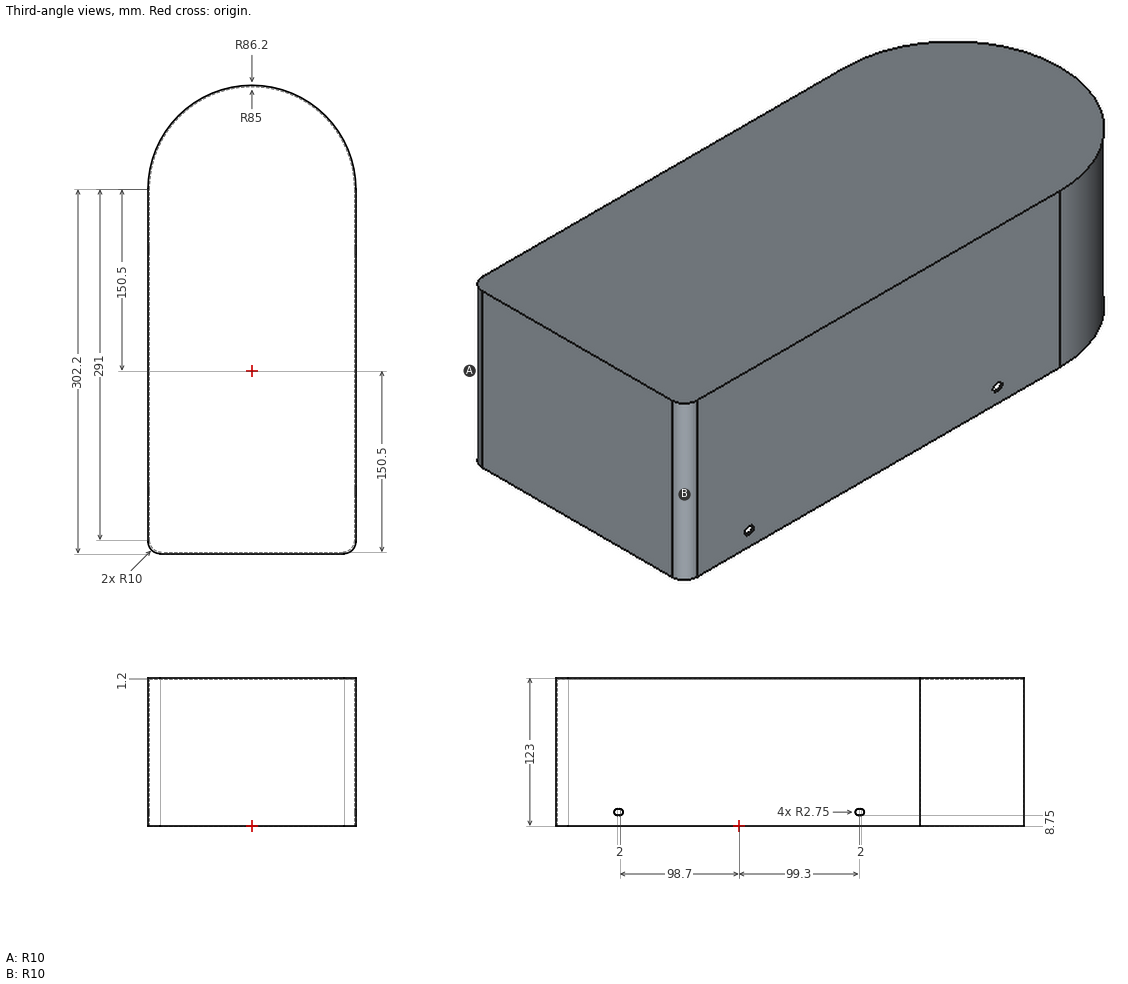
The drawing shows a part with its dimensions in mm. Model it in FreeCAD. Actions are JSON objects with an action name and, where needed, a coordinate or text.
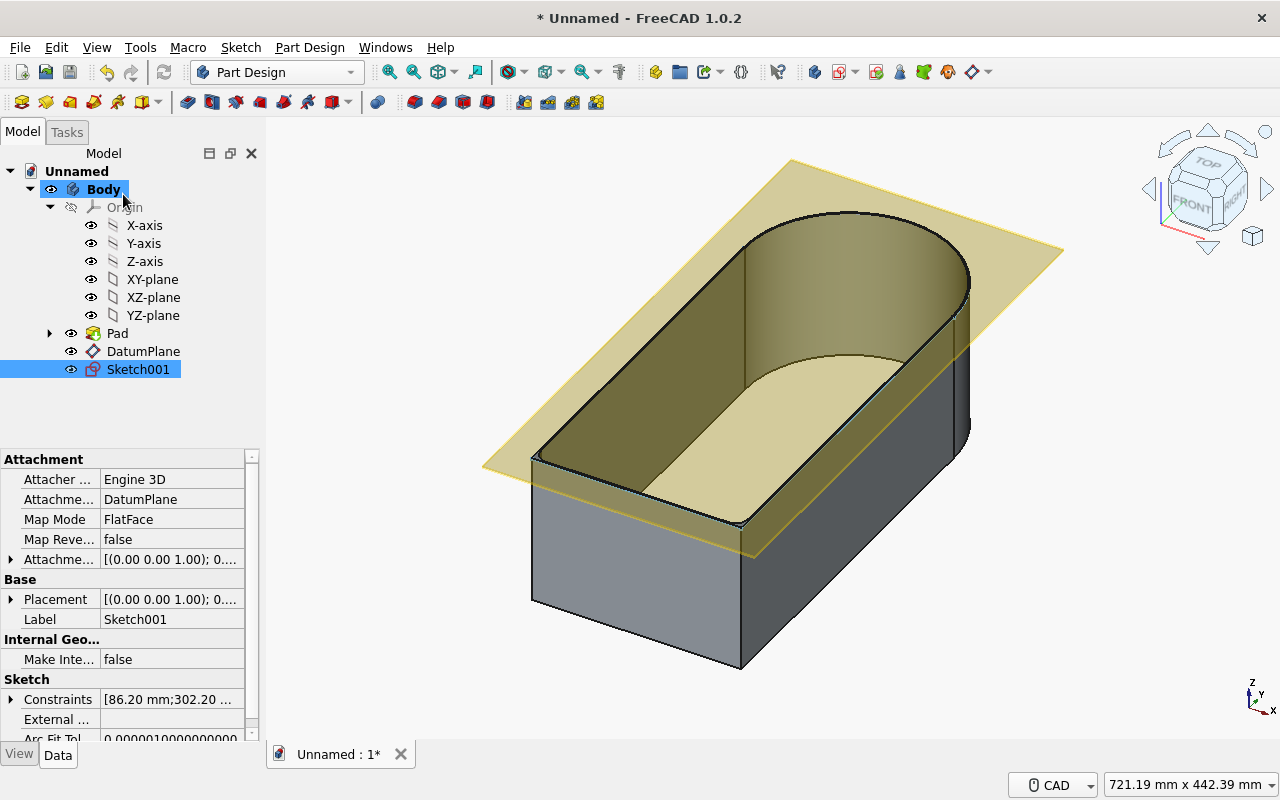
{"action": "left_click", "coordinate": [22, 102]}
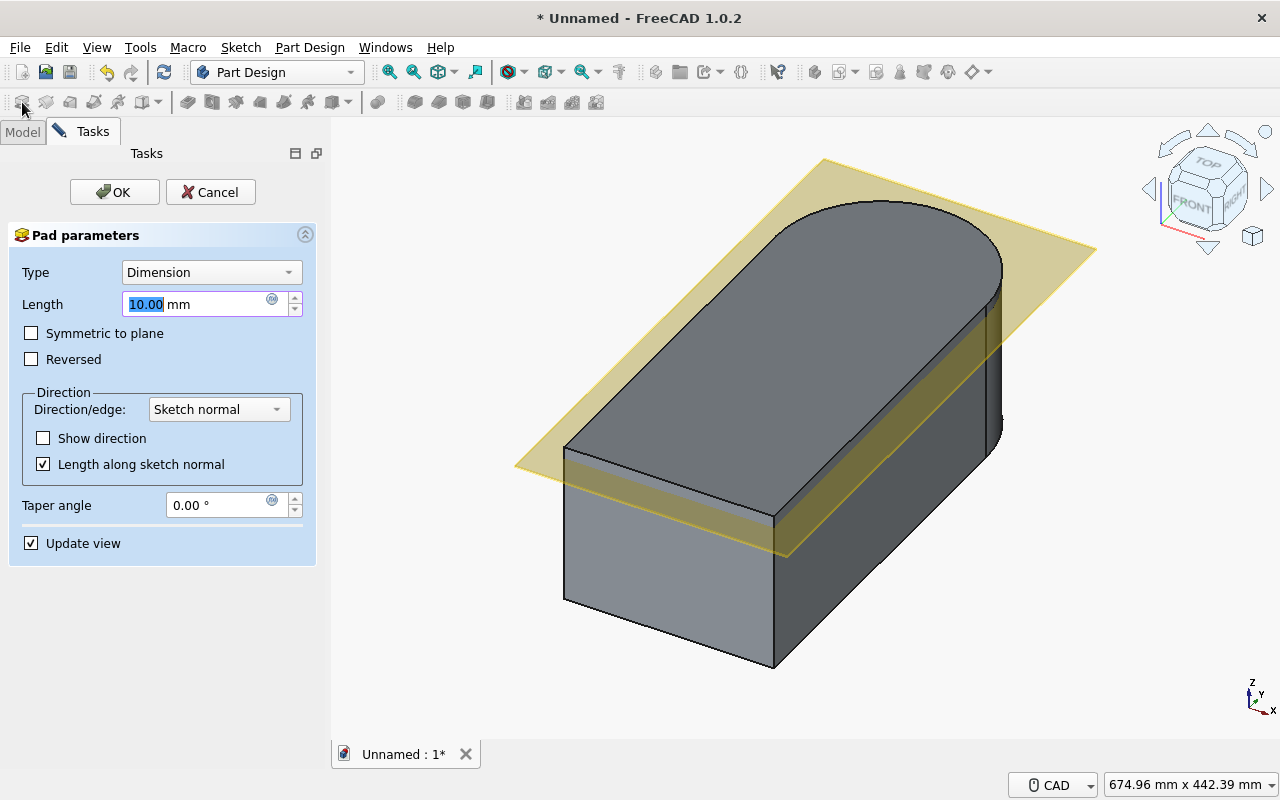
{"action": "type", "text": "1.2"}
{"action": "key", "text": "Tab"}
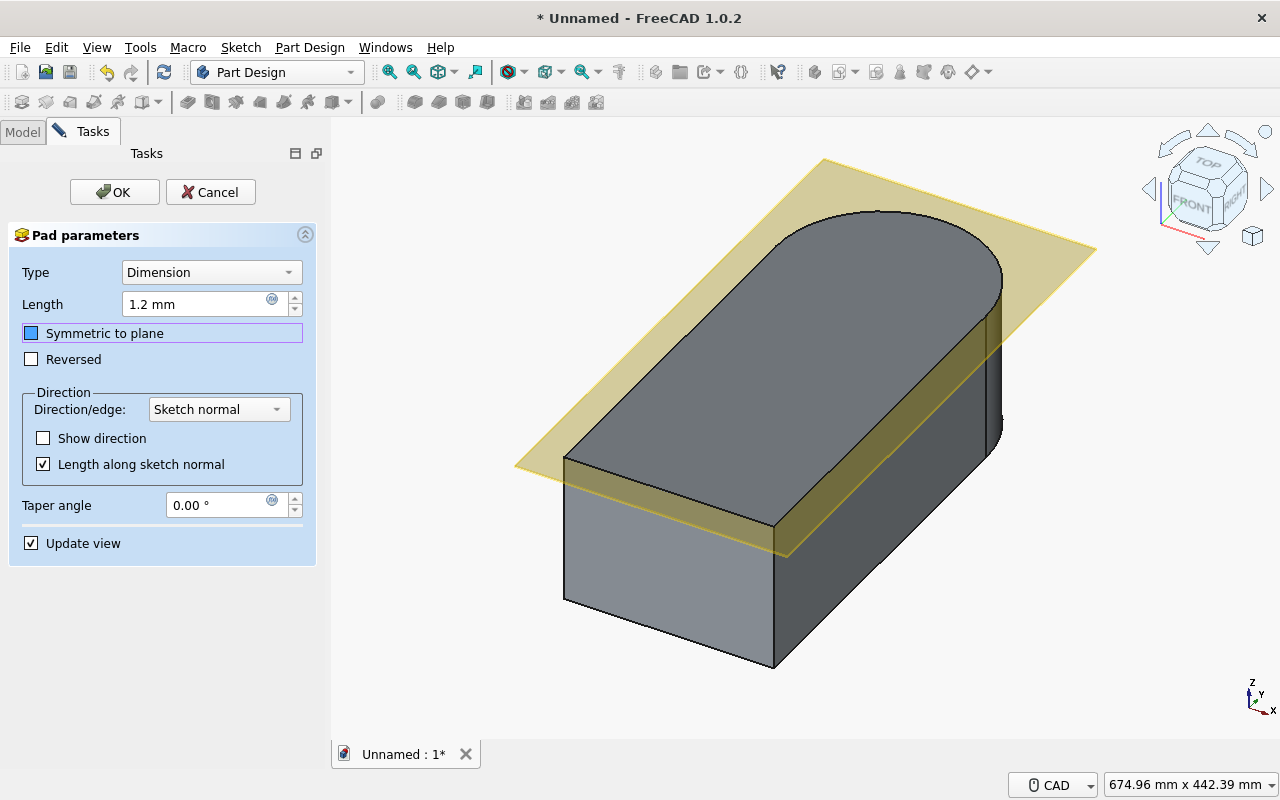
{"action": "left_click", "coordinate": [115, 192]}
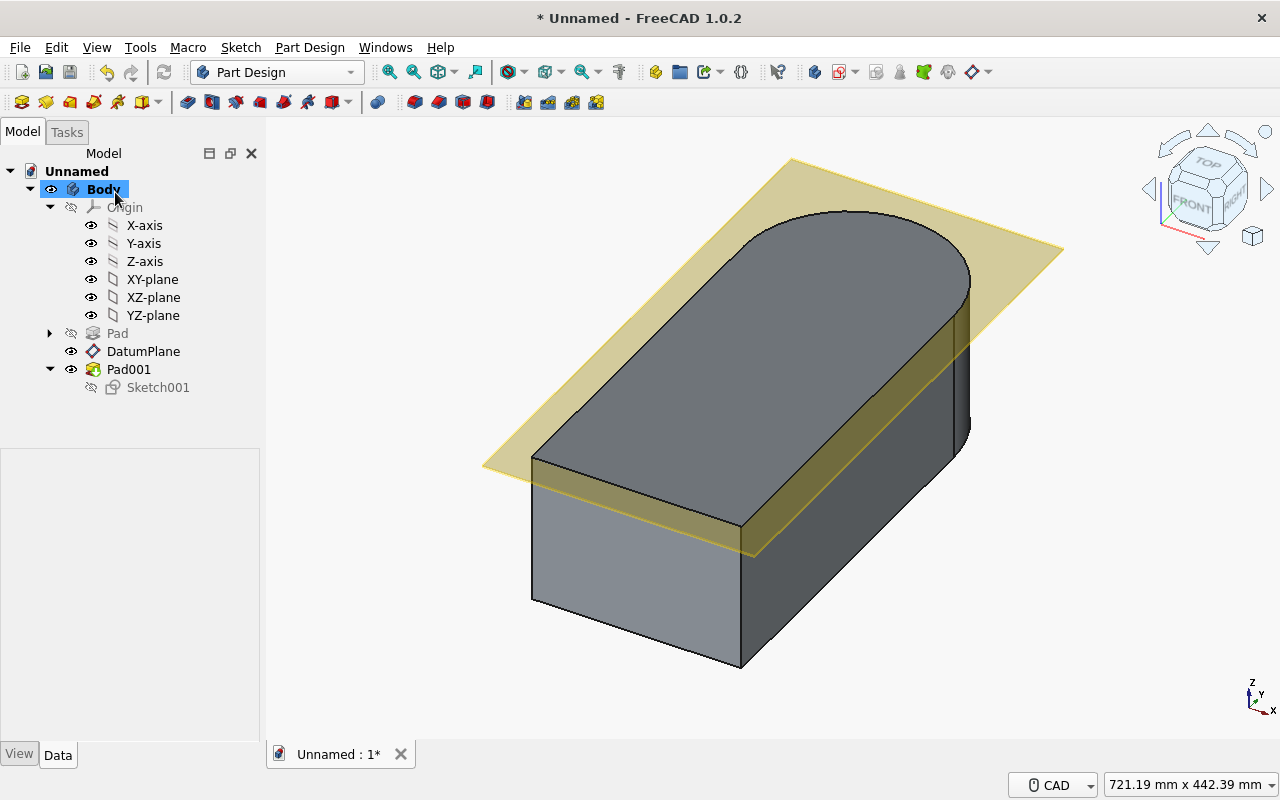
{"action": "left_click", "coordinate": [116, 351]}
{"action": "key", "text": "space"}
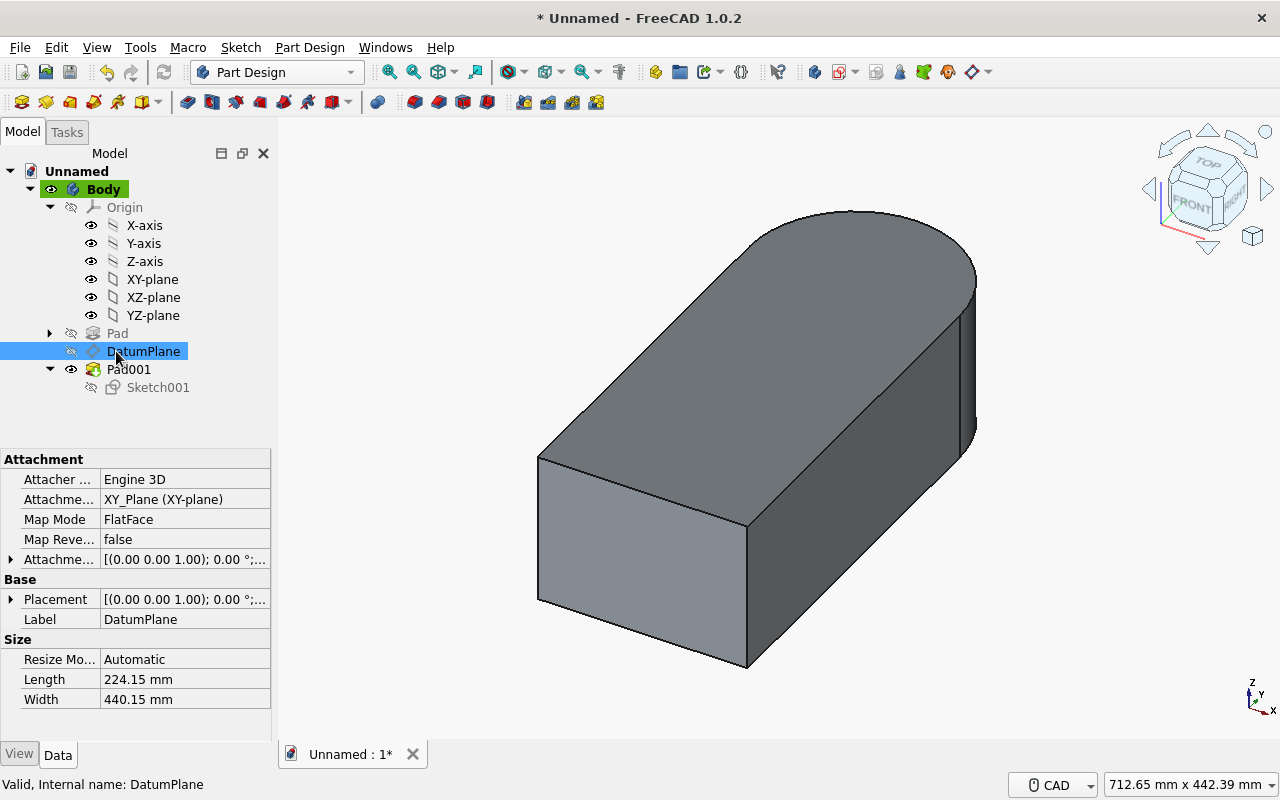
{"action": "key", "text": "0"}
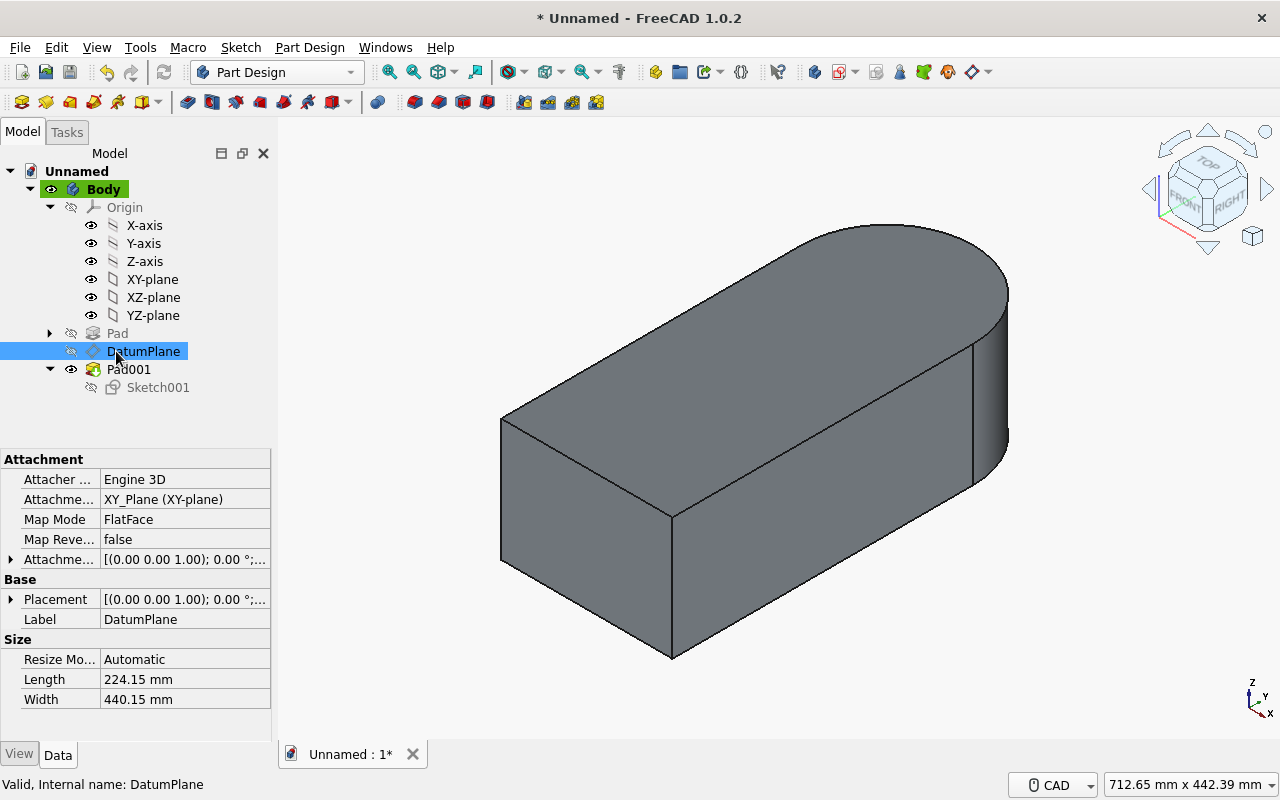
{"action": "key", "text": "2"}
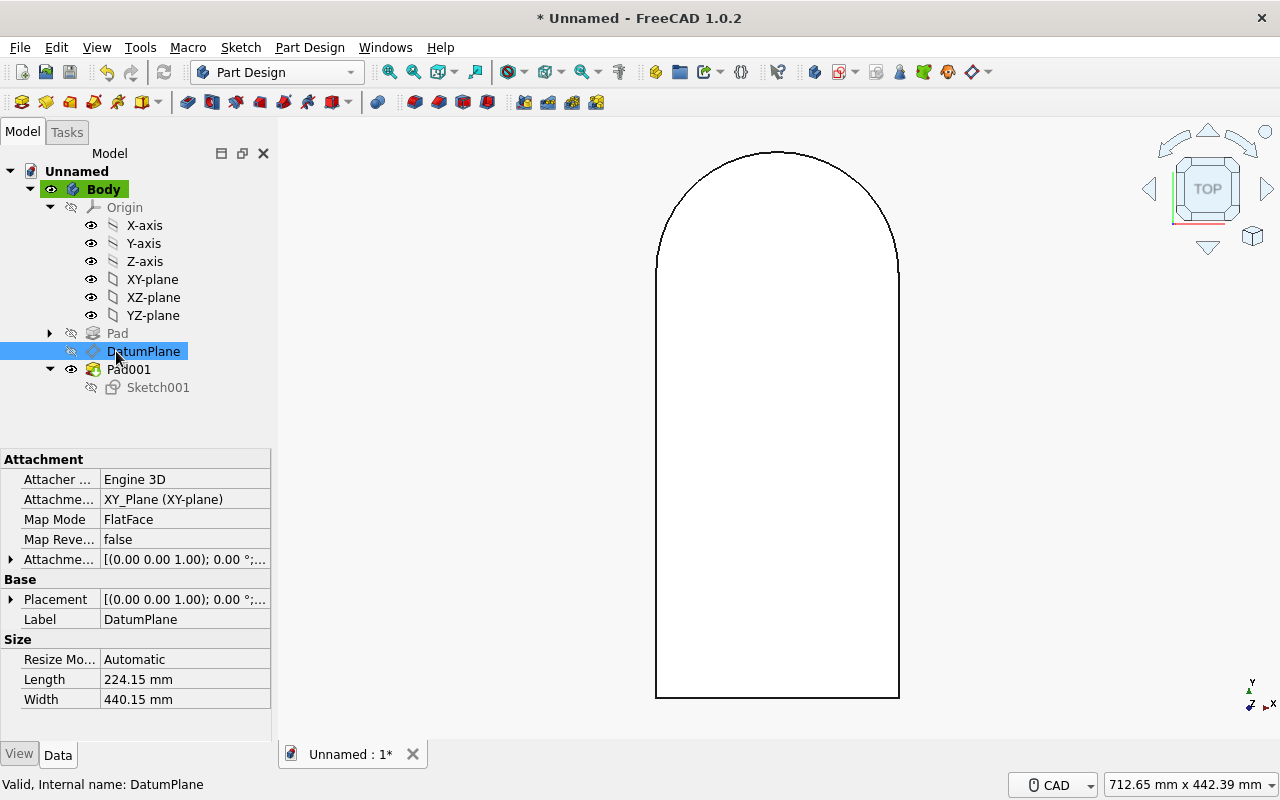
{"action": "key", "text": "1"}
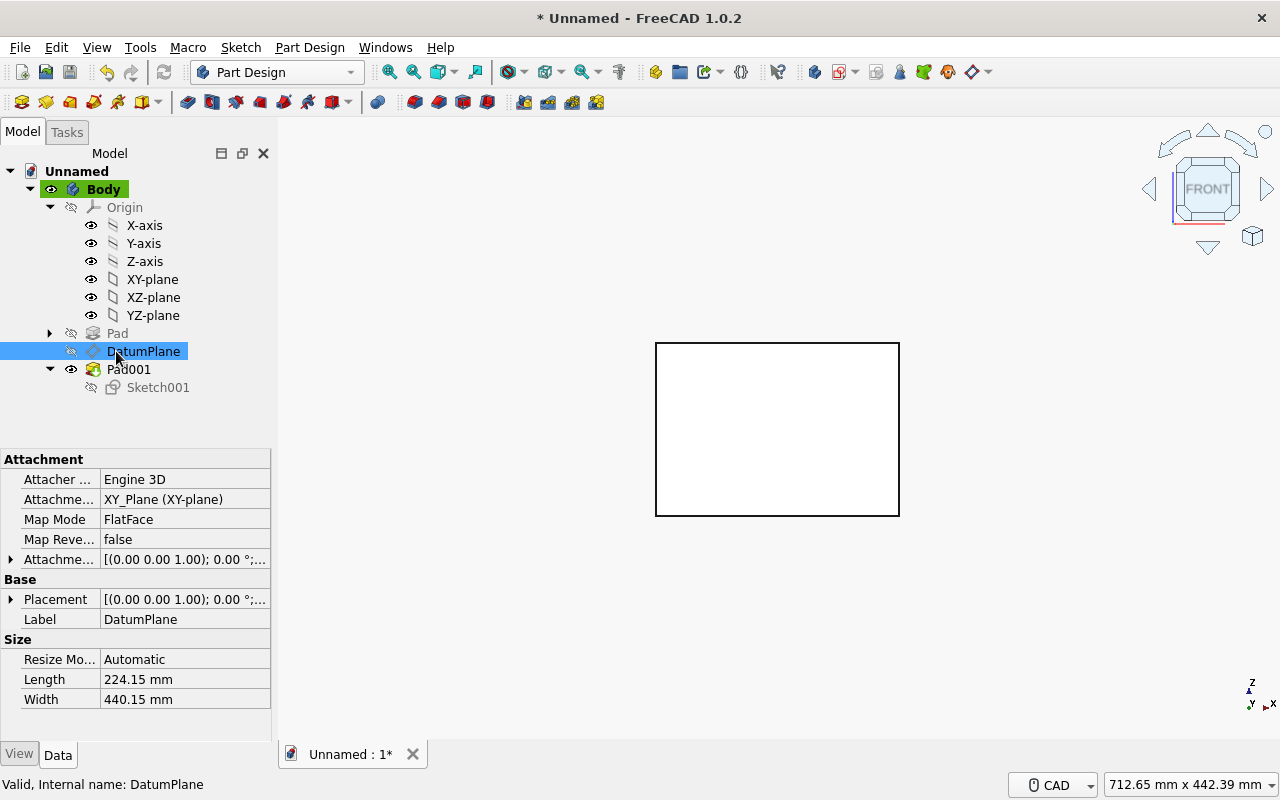
{"action": "key", "text": "v f"}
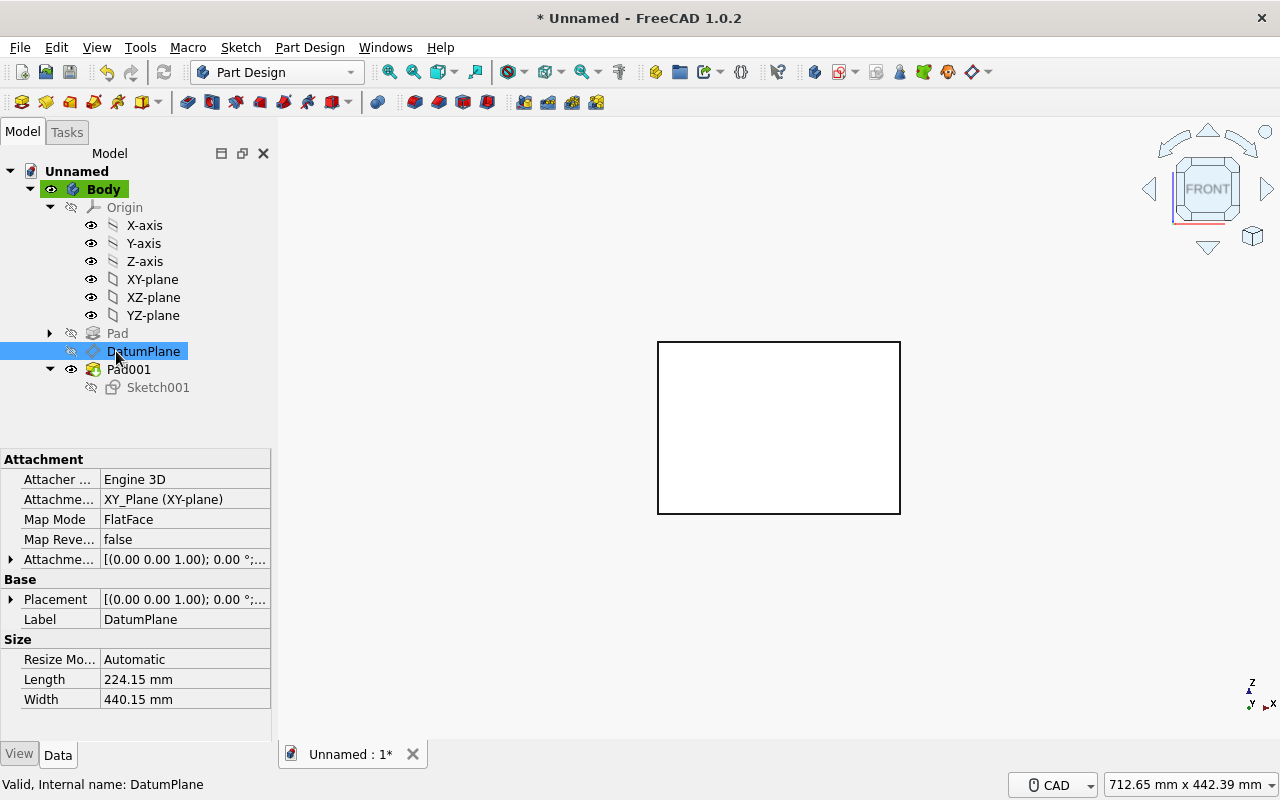
{"action": "left_click", "coordinate": [658, 427]}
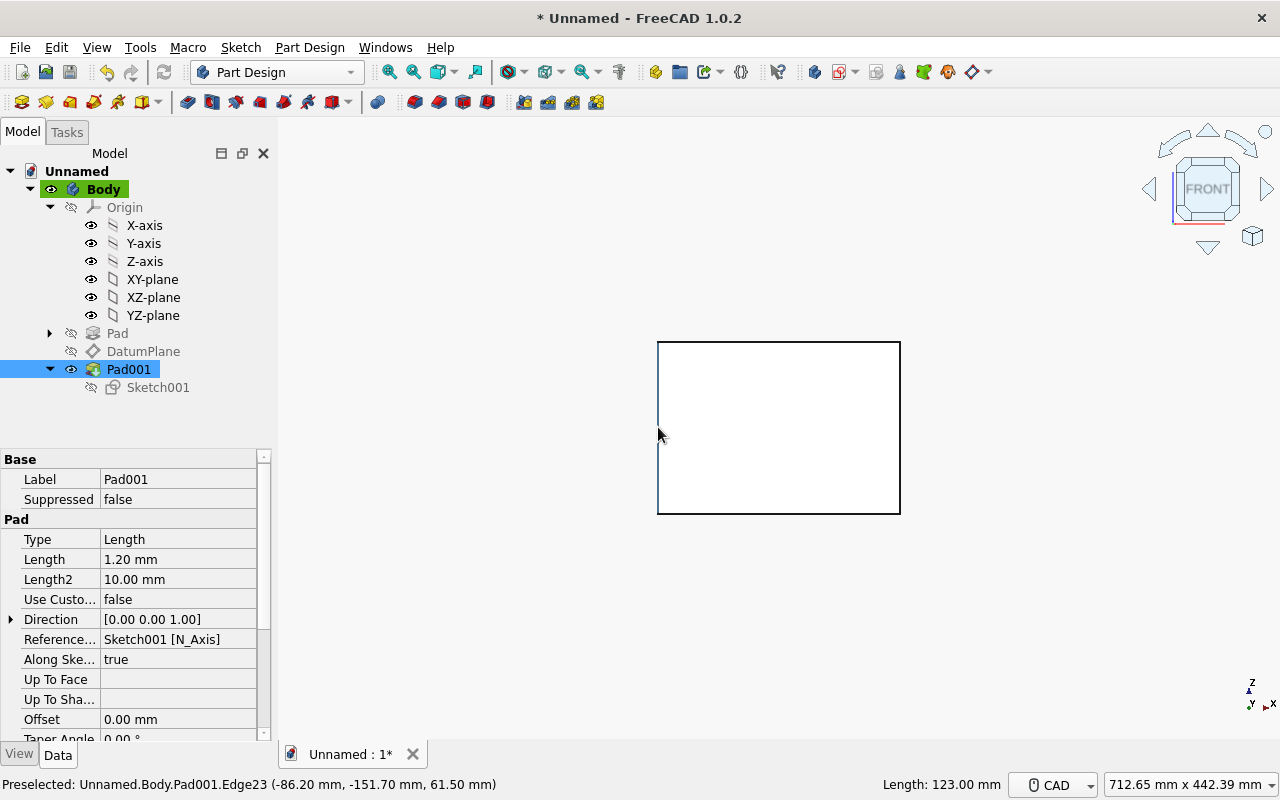
{"action": "left_click", "coordinate": [416, 102]}